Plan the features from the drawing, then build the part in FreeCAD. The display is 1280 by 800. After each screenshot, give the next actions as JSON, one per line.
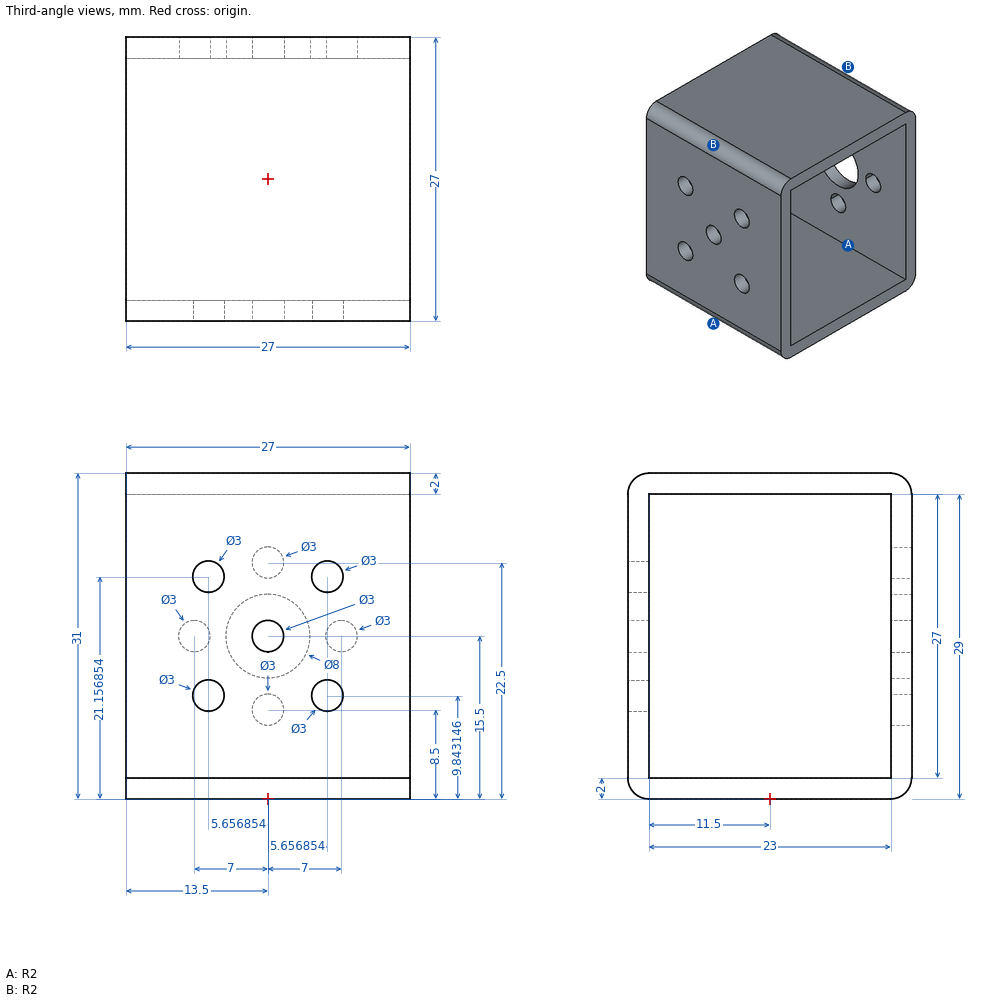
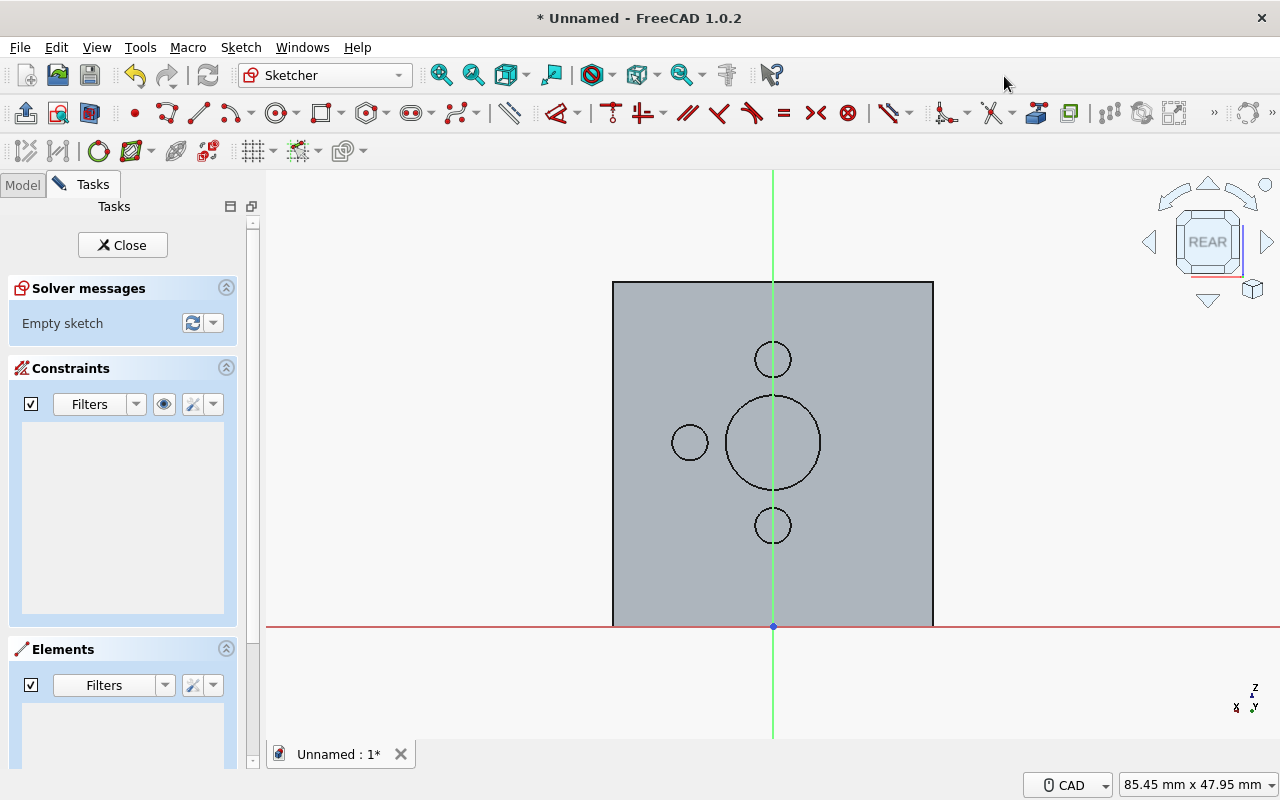
{"action": "scroll", "coordinate": [871, 441], "scroll_direction": "up", "scroll_amount": 12}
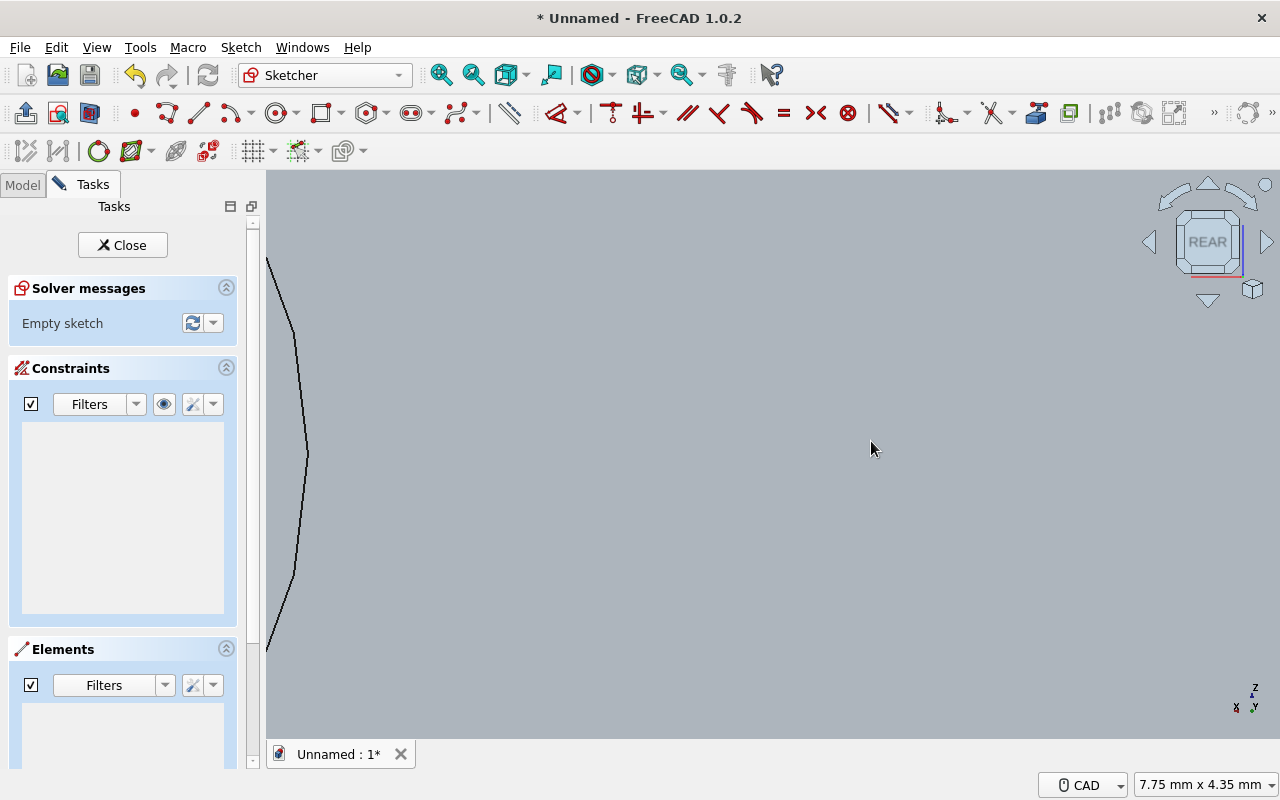
{"action": "left_click", "coordinate": [276, 114]}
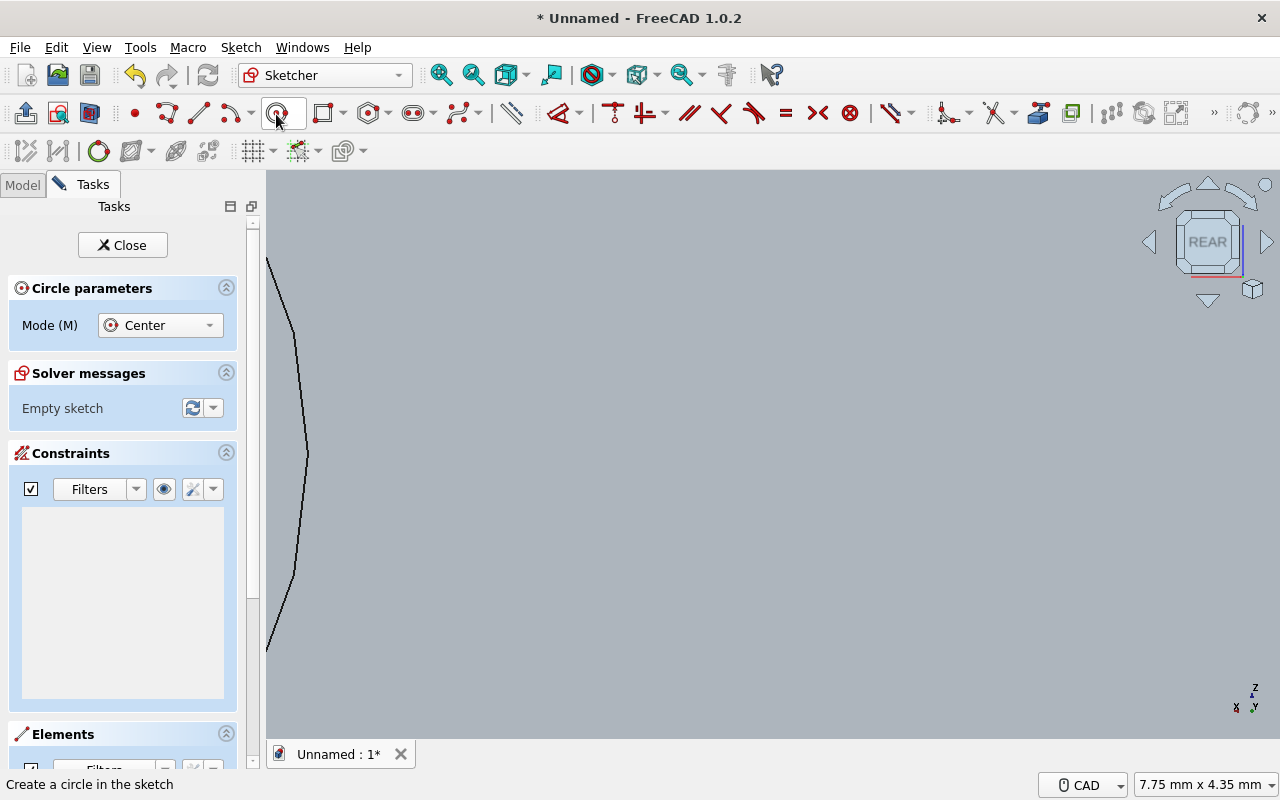
{"action": "left_click", "coordinate": [700, 454]}
{"action": "mouse_move", "coordinate": [839, 315]}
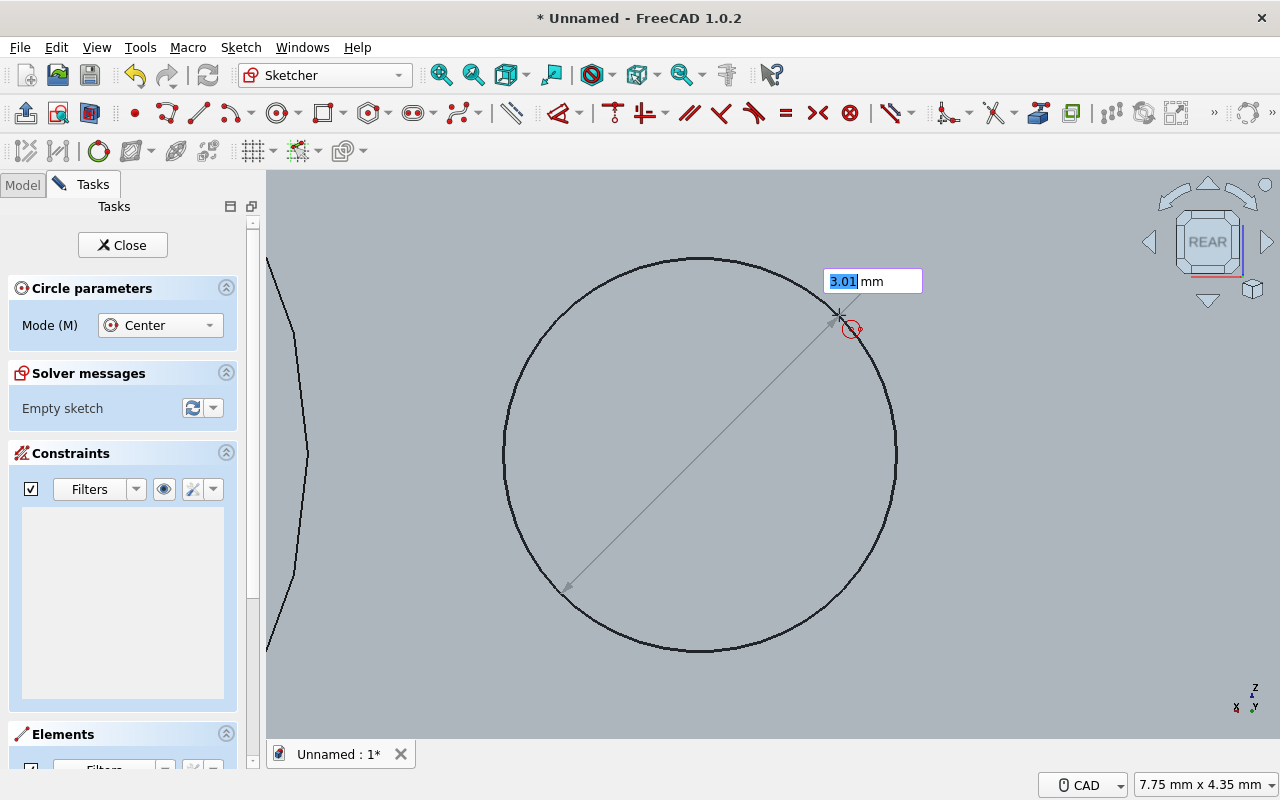
{"action": "type", "text": "3"}
{"action": "key", "text": "Return"}
{"action": "key", "text": "Escape"}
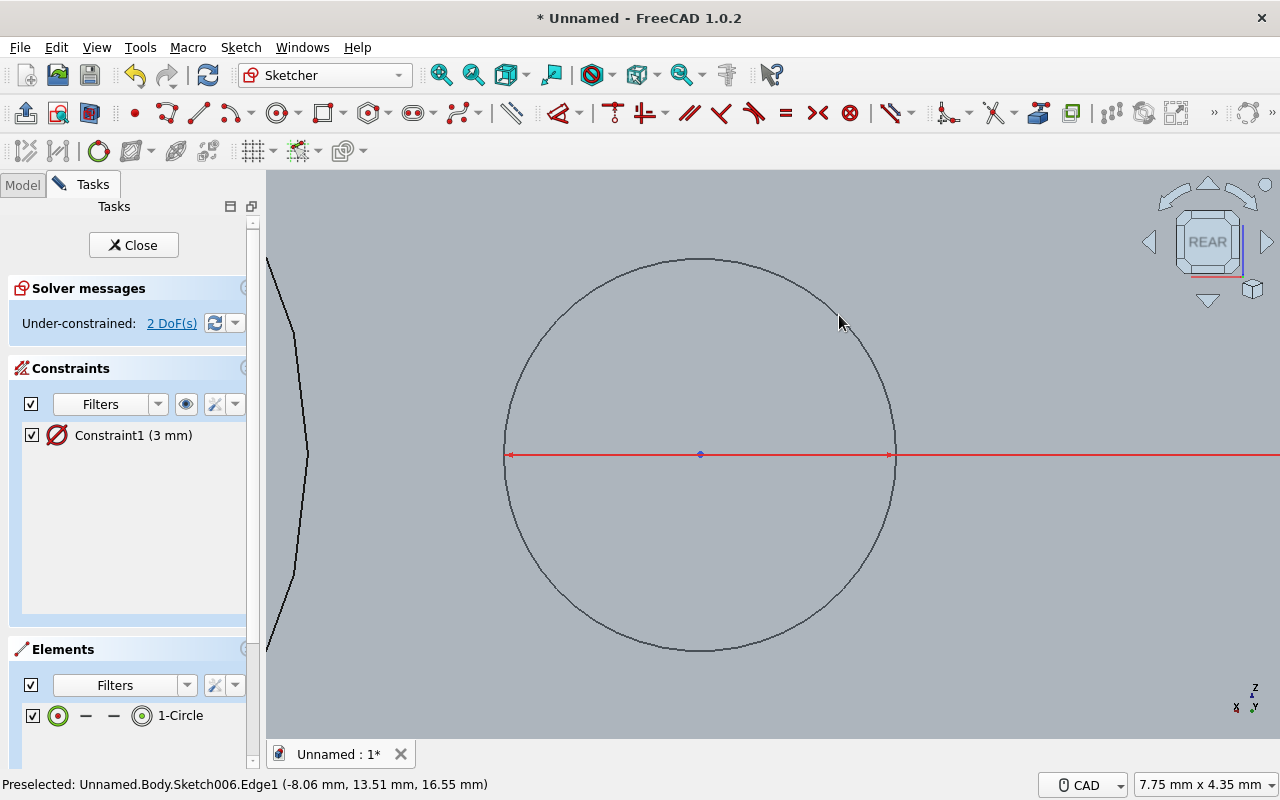
{"action": "left_click", "coordinate": [558, 114]}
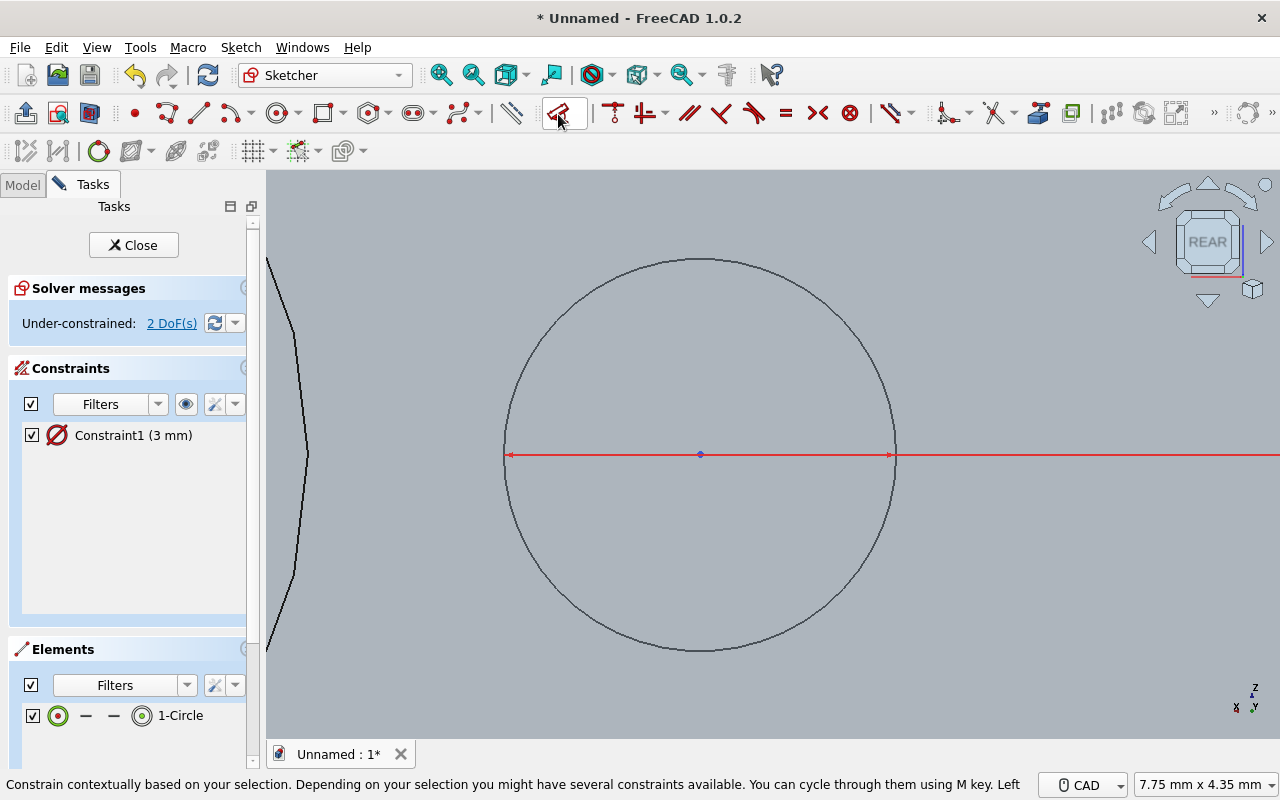
{"action": "left_click", "coordinate": [700, 455]}
{"action": "left_click", "coordinate": [404, 421]}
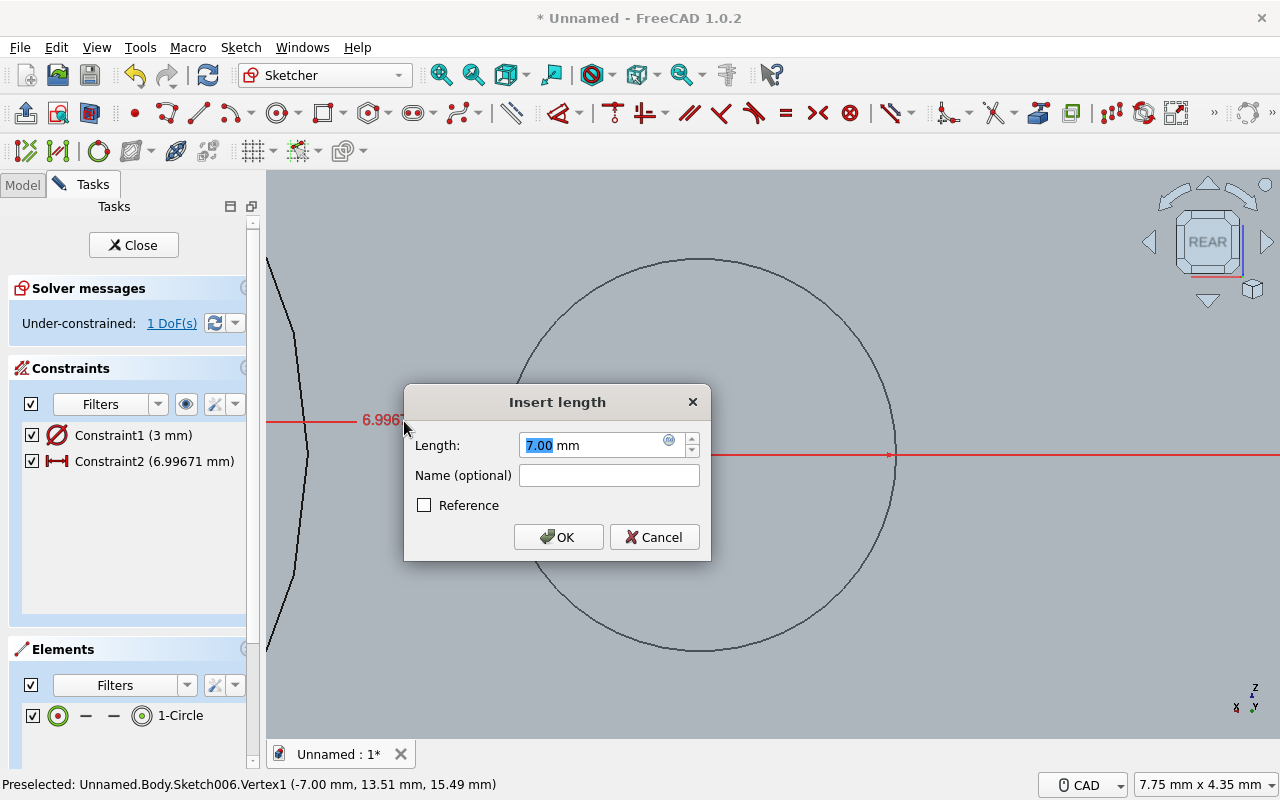
{"action": "type", "text": "7"}
{"action": "key", "text": "Return"}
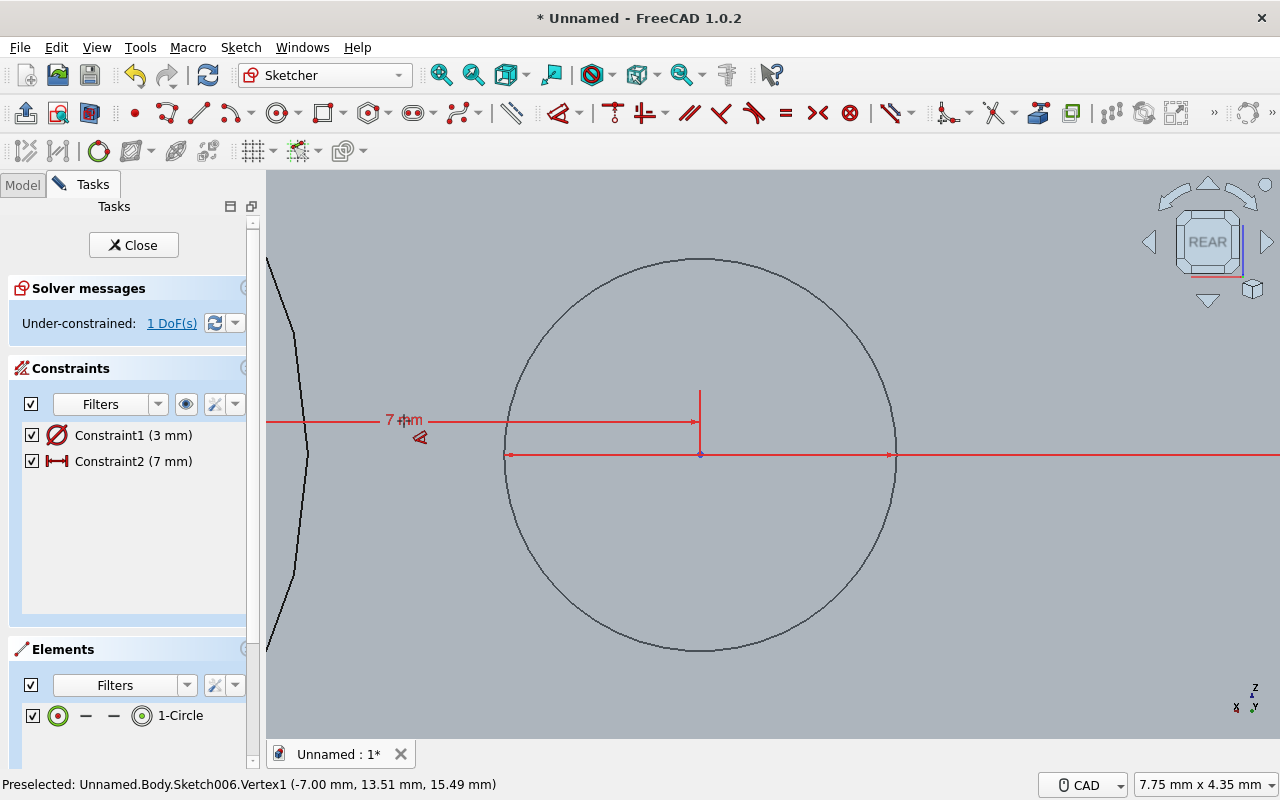
{"action": "left_click", "coordinate": [700, 455]}
{"action": "left_click", "coordinate": [734, 583]}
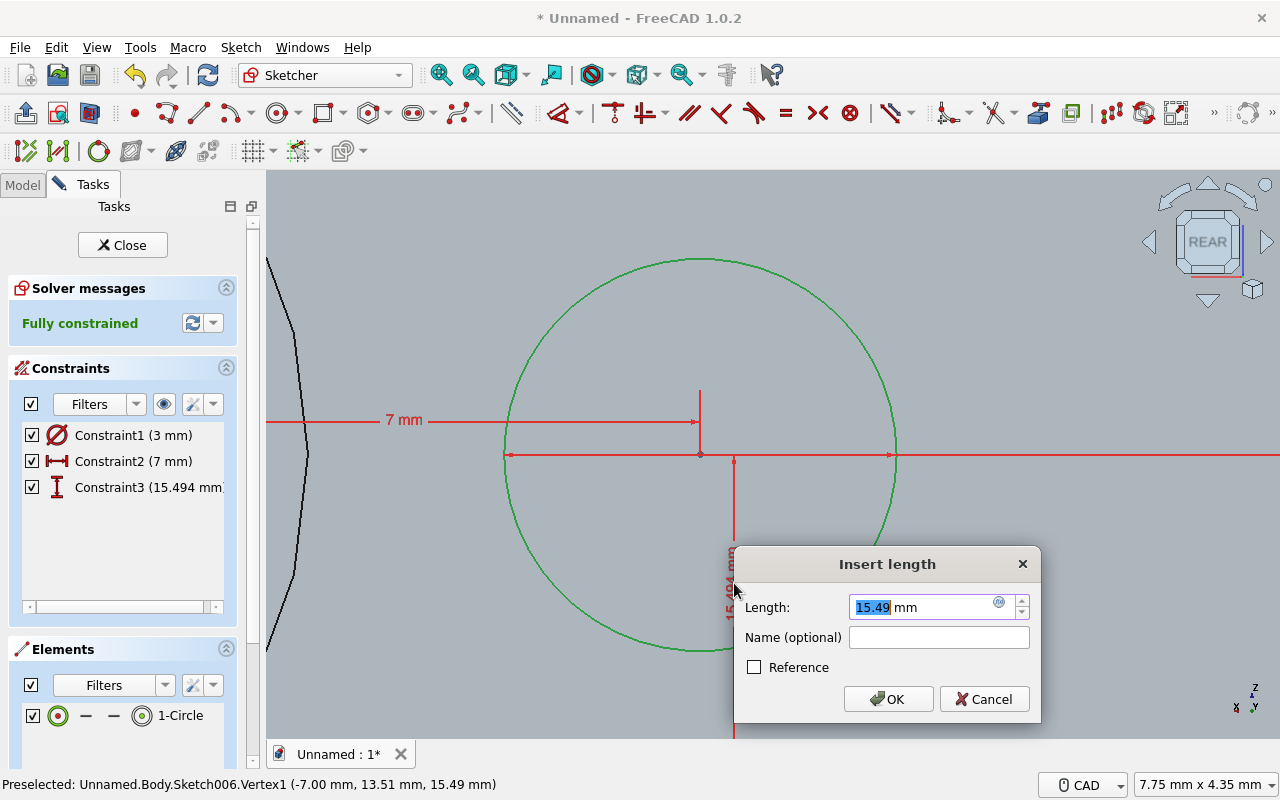
{"action": "type", "text": "15.5"}
{"action": "key", "text": "Return"}
{"action": "key", "text": "Escape"}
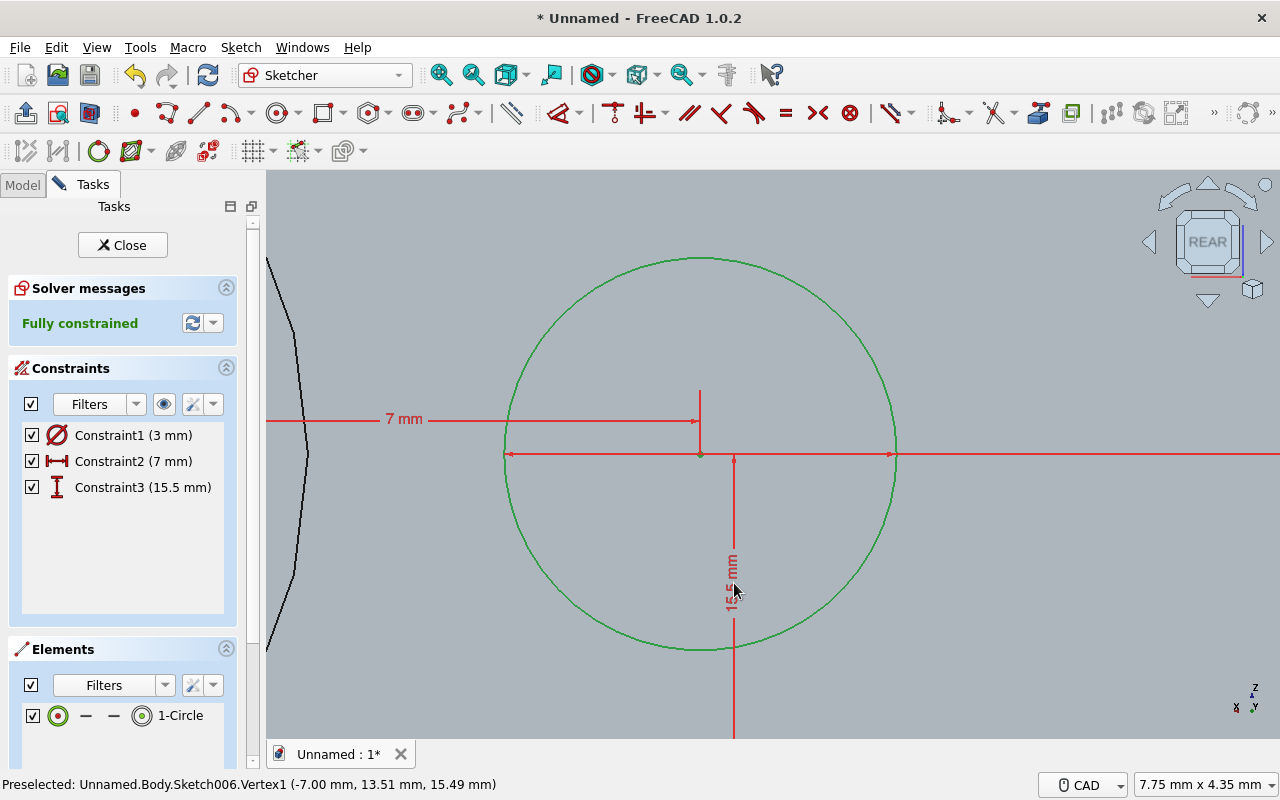
{"action": "left_click", "coordinate": [123, 245]}